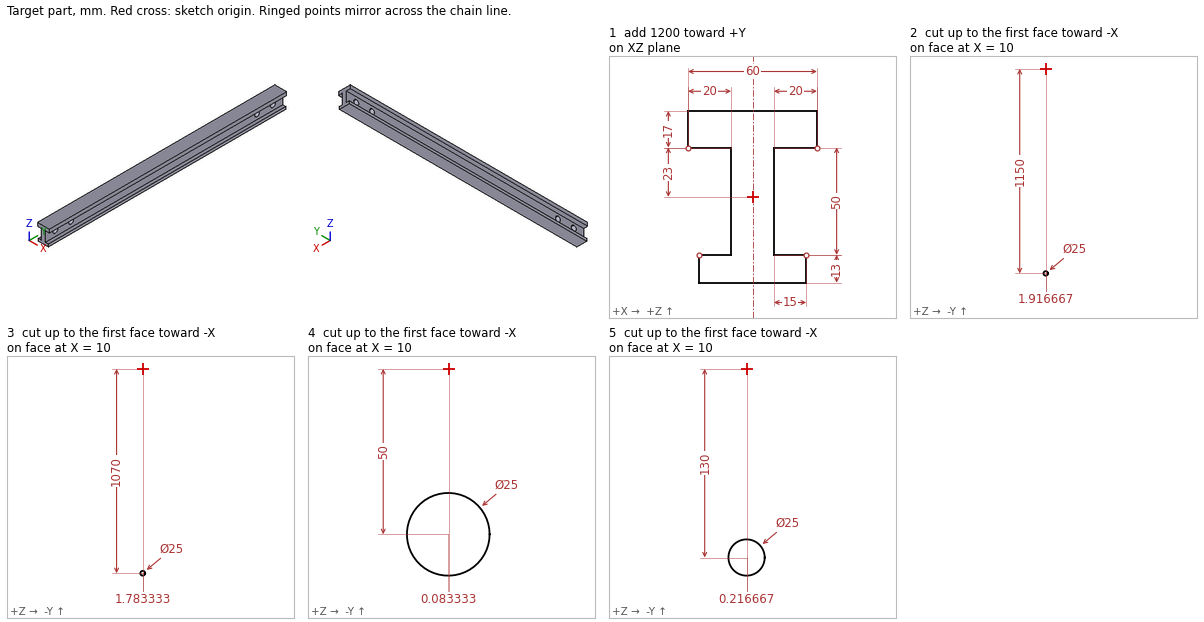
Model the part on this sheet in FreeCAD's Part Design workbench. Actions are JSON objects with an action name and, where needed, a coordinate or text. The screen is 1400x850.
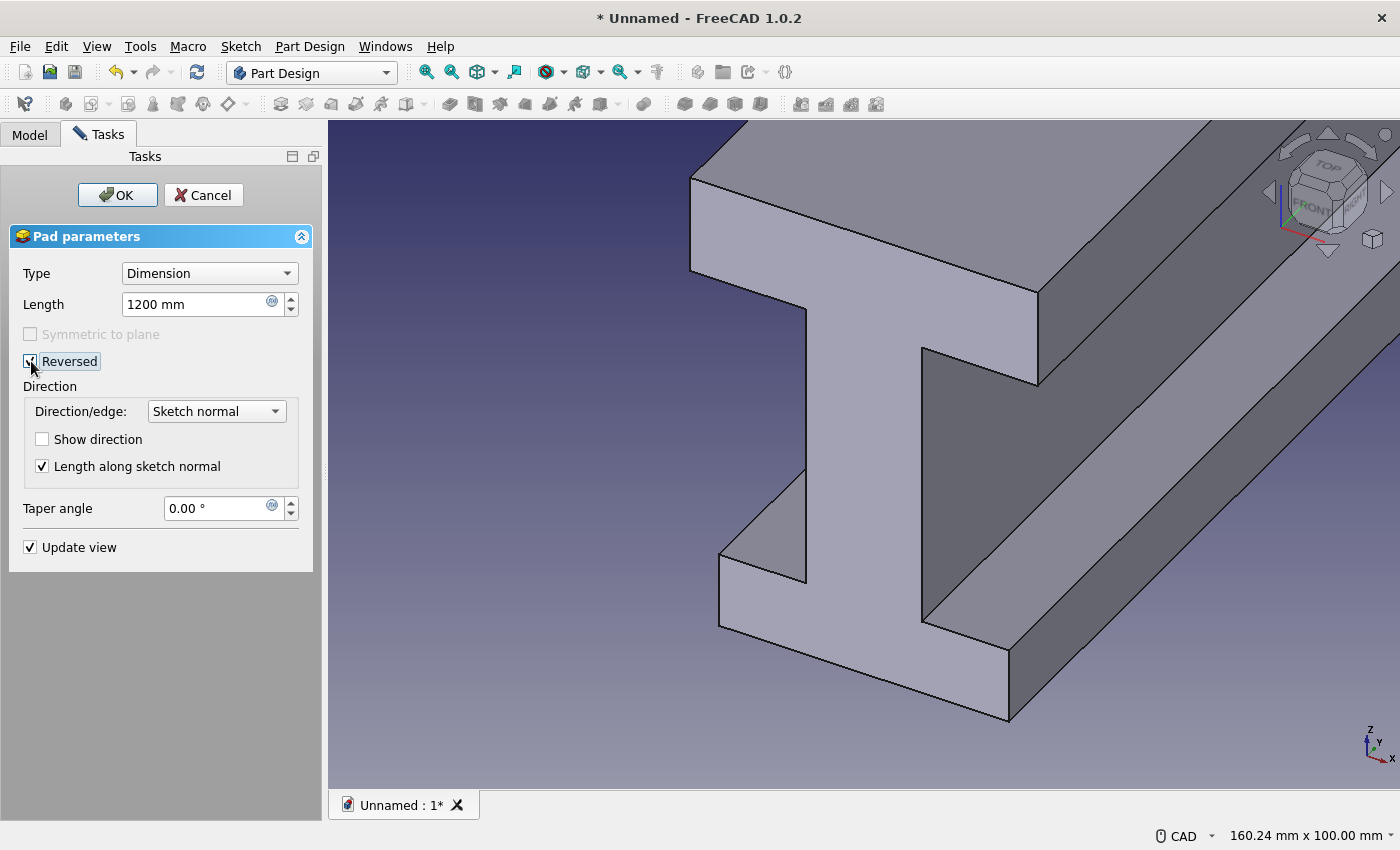
{"action": "left_click", "coordinate": [118, 195]}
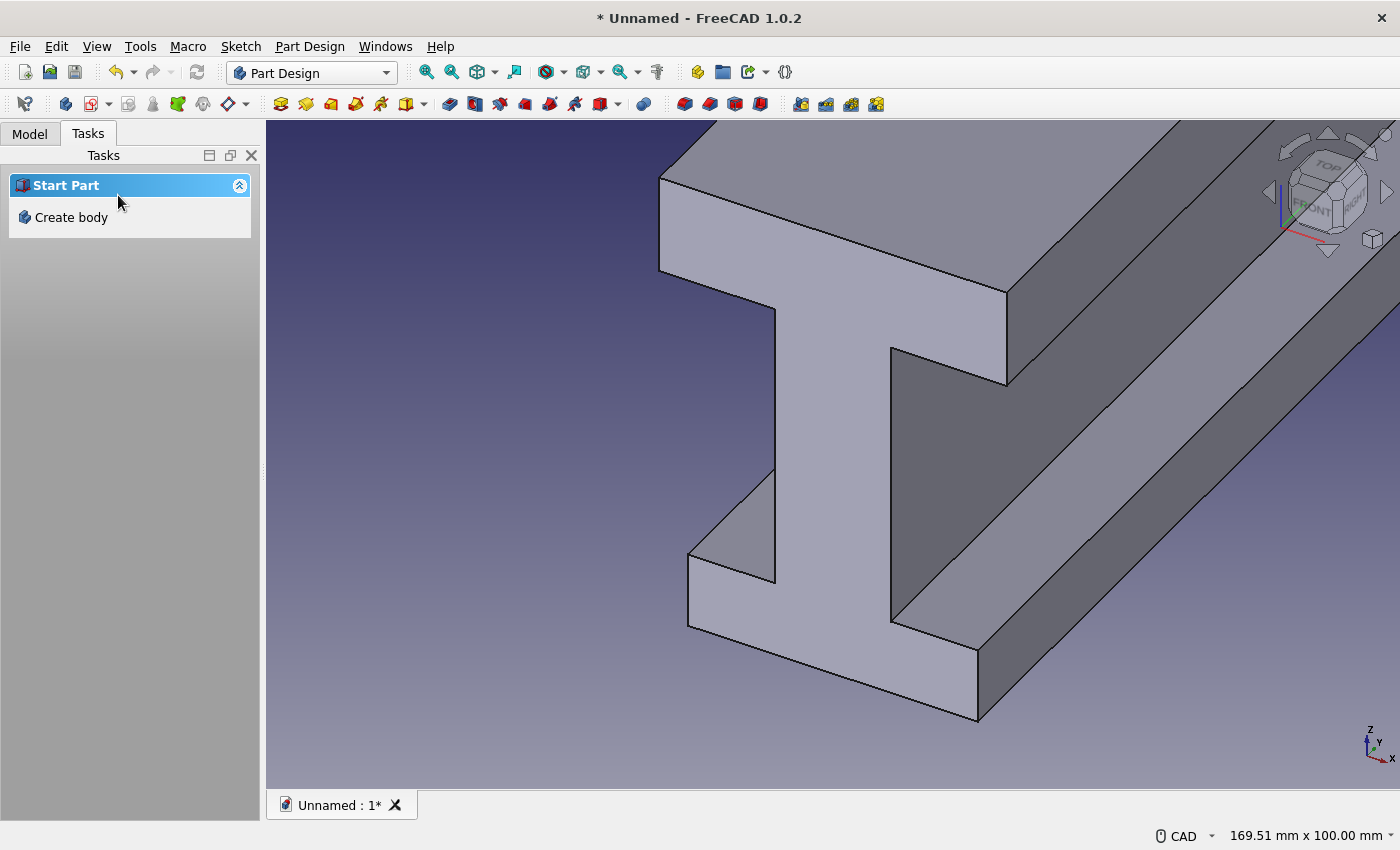
{"action": "left_click", "coordinate": [427, 72]}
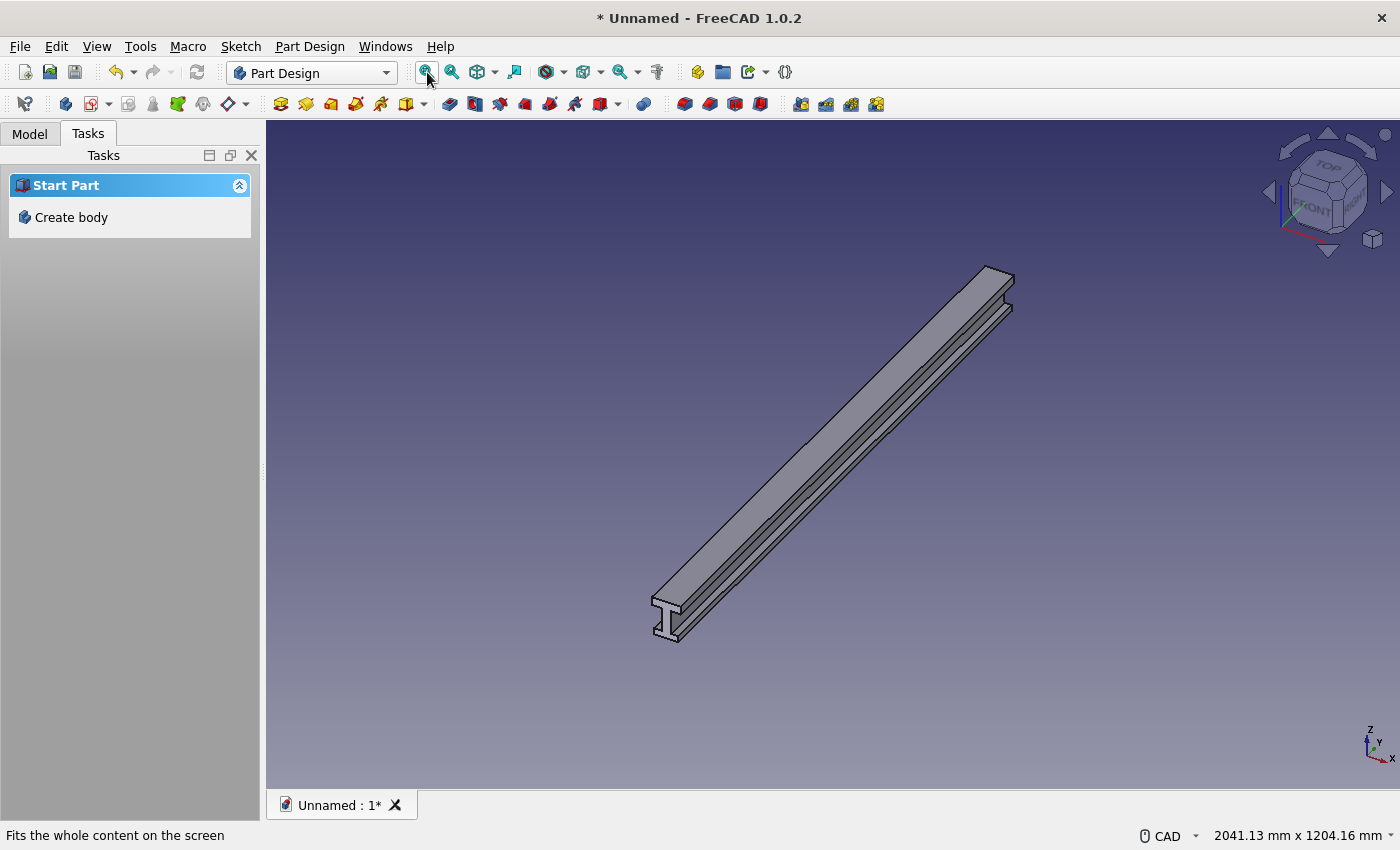
{"action": "key", "text": "0"}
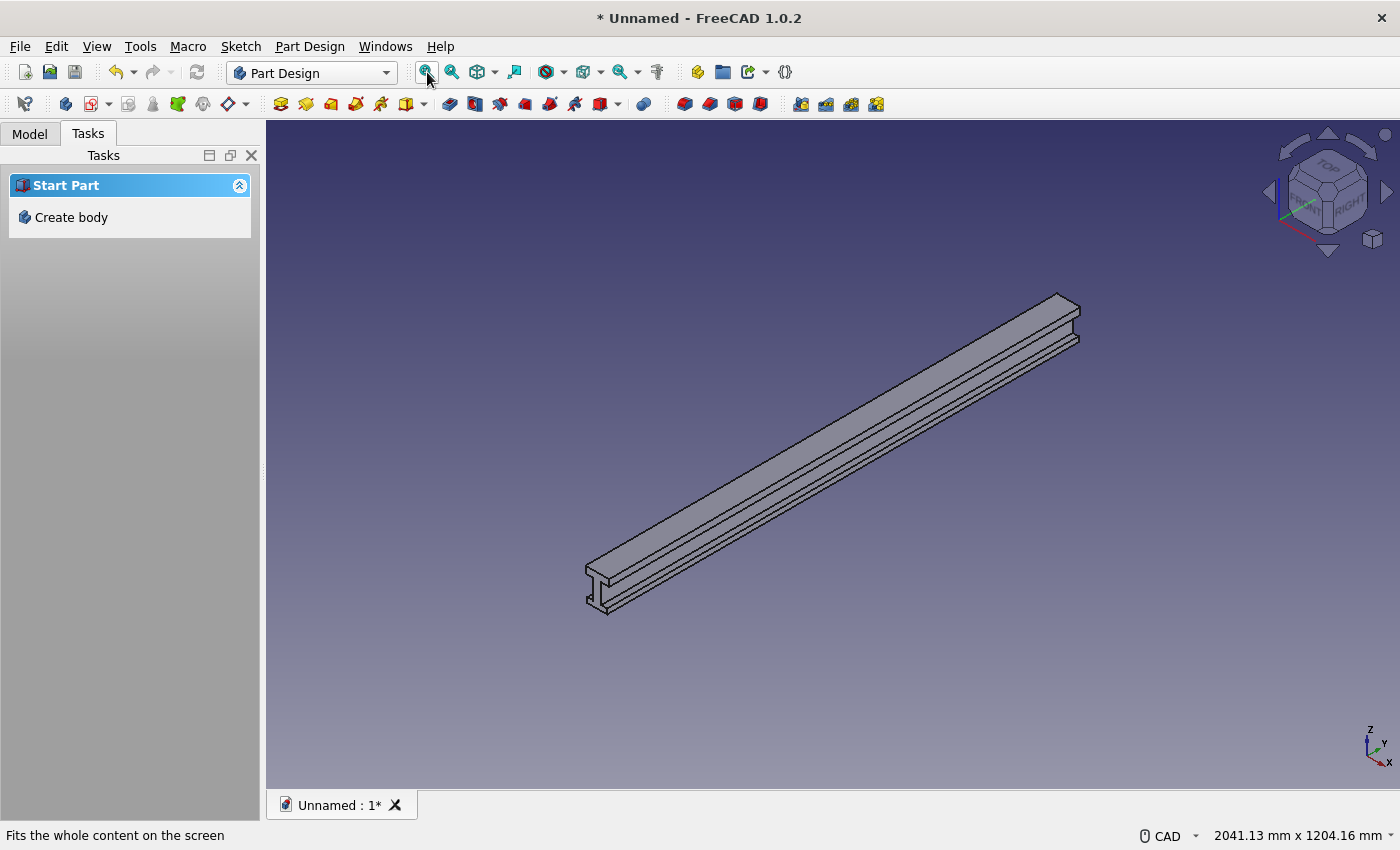
{"action": "key", "text": "3"}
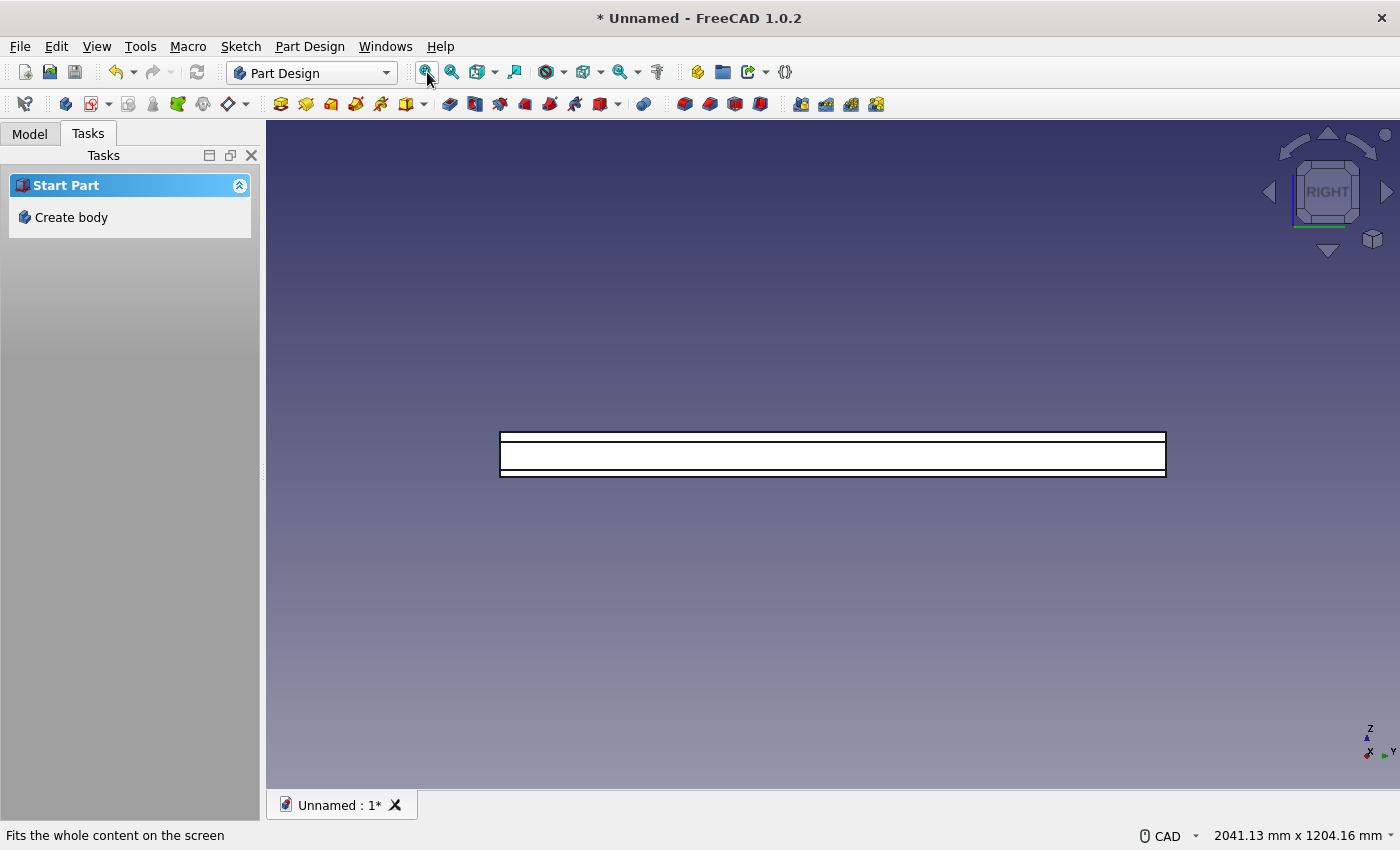
{"action": "left_click", "coordinate": [1023, 455]}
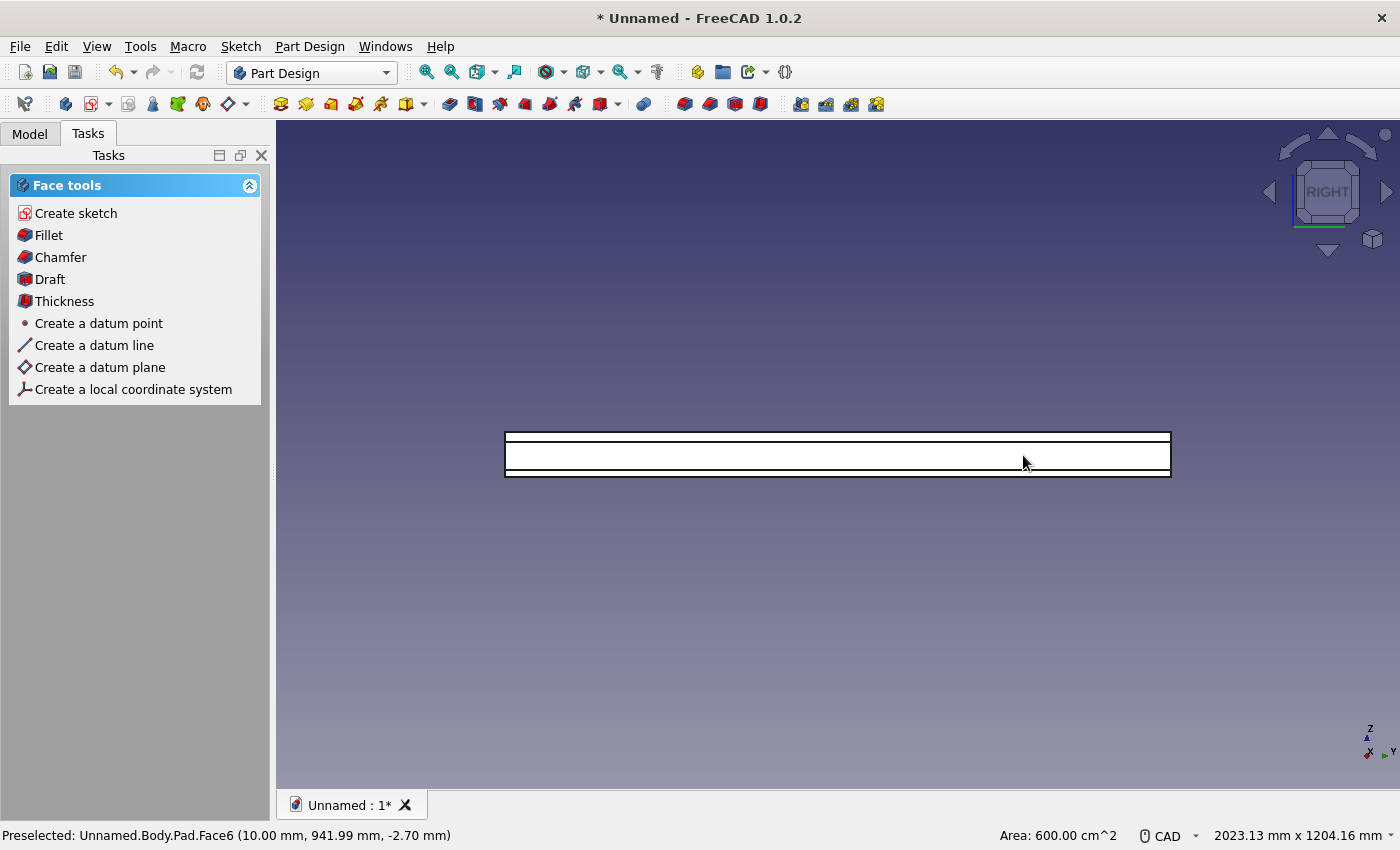
{"action": "left_click", "coordinate": [90, 104]}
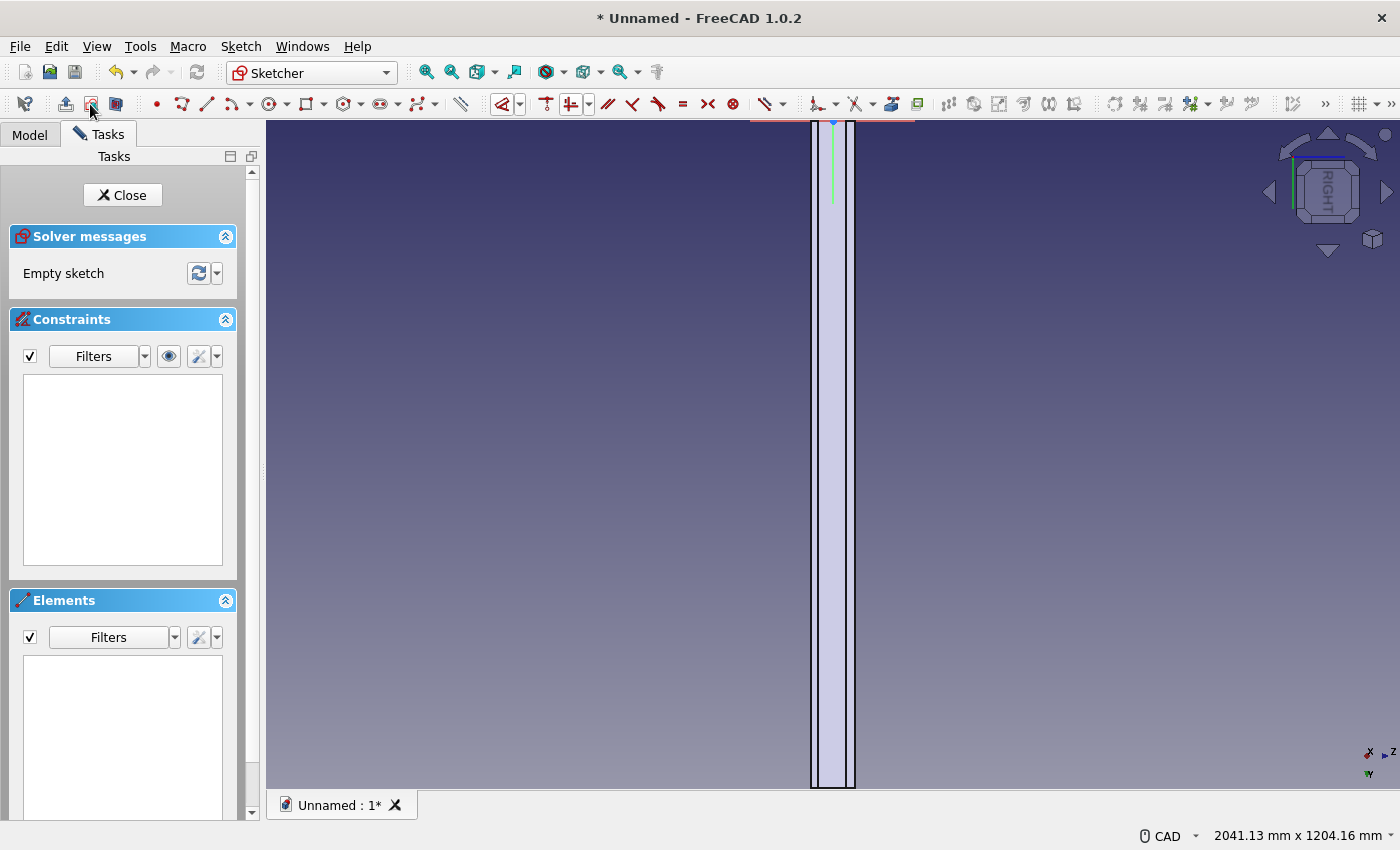
{"action": "left_click", "coordinate": [116, 104]}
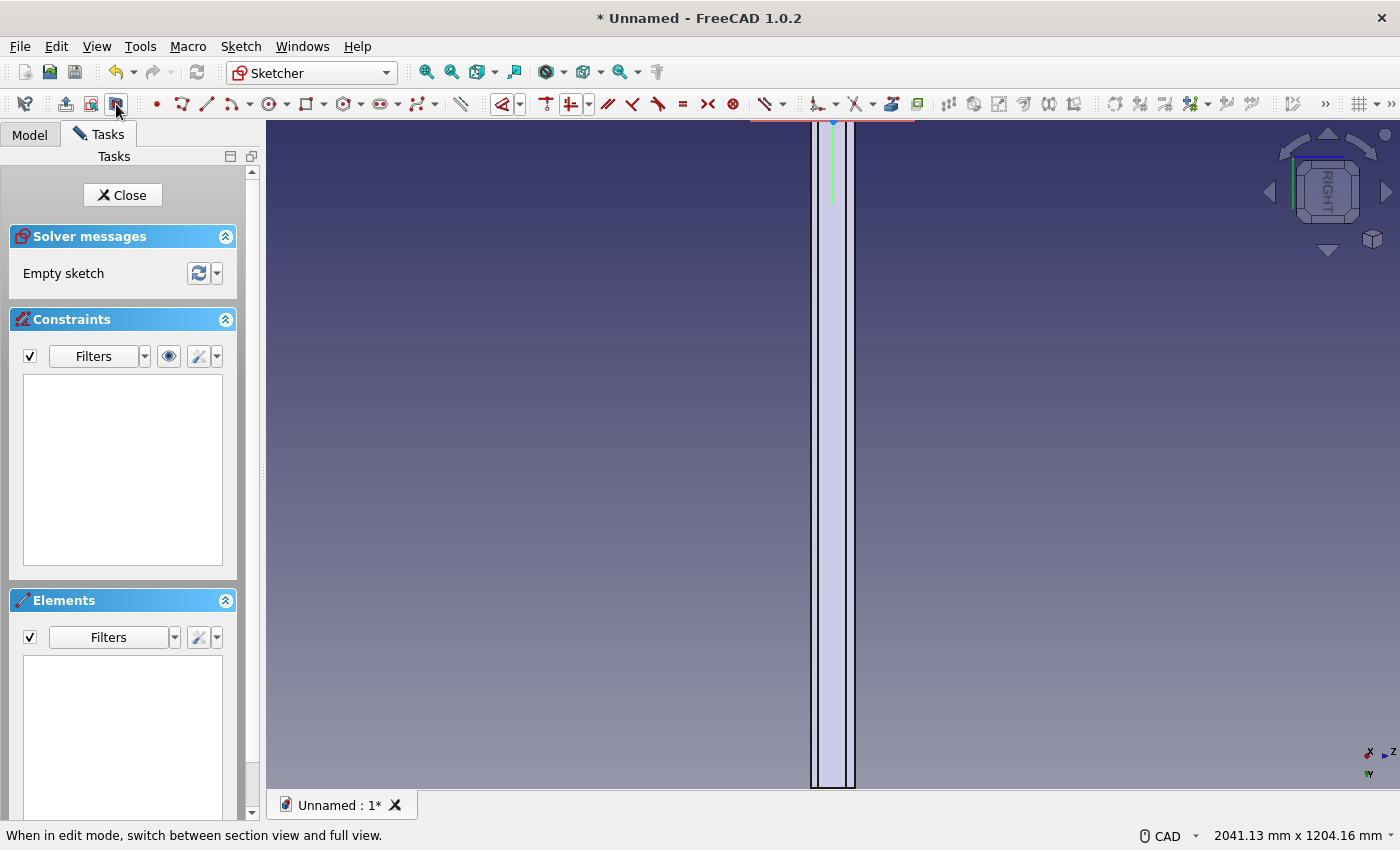
{"action": "scroll", "coordinate": [764, 454], "scroll_direction": "down", "scroll_amount": 5}